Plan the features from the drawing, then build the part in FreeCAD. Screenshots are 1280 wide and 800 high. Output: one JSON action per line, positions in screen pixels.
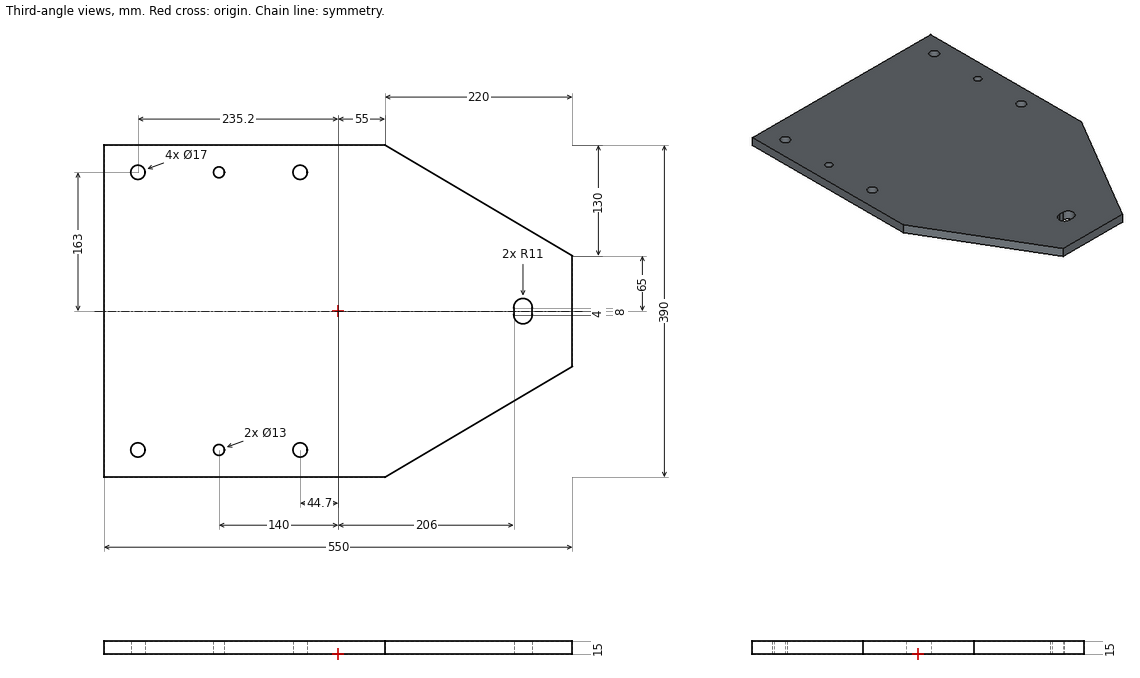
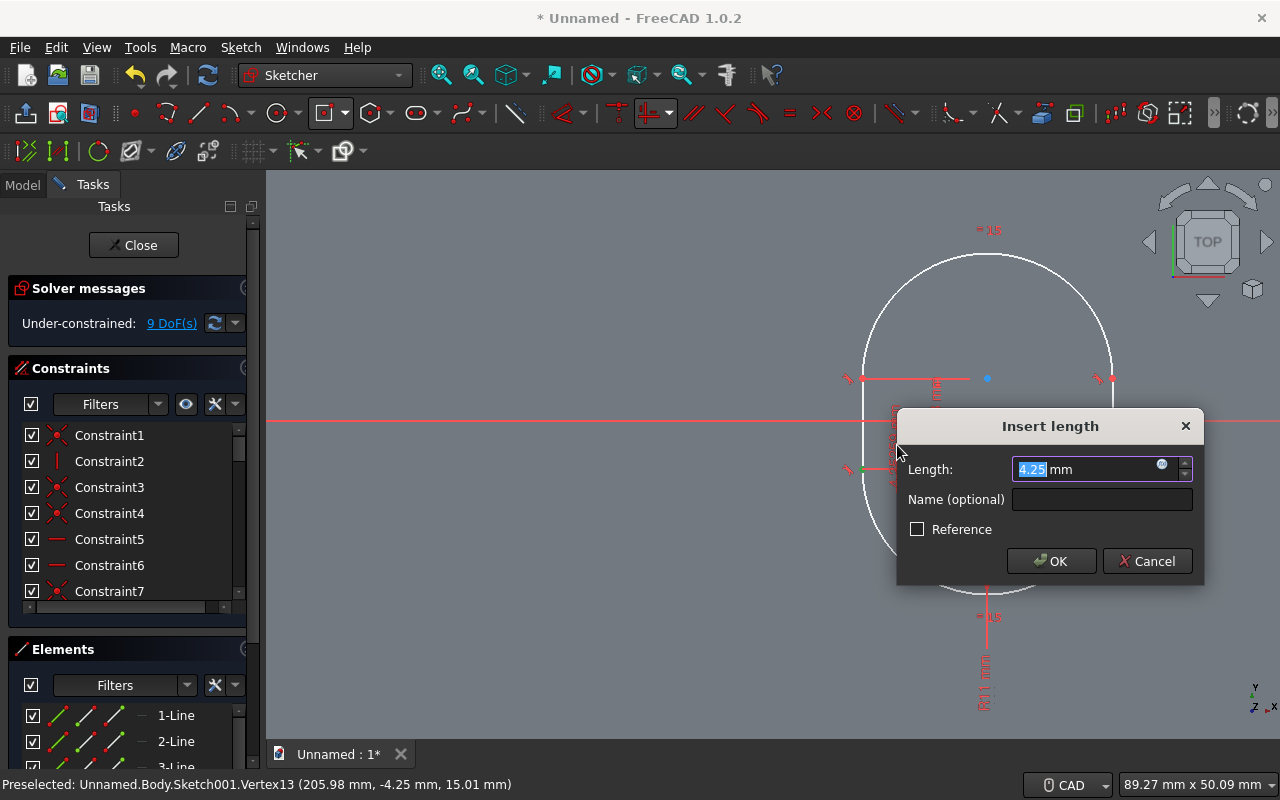
{"action": "type", "text": "4"}
{"action": "key", "text": "Return"}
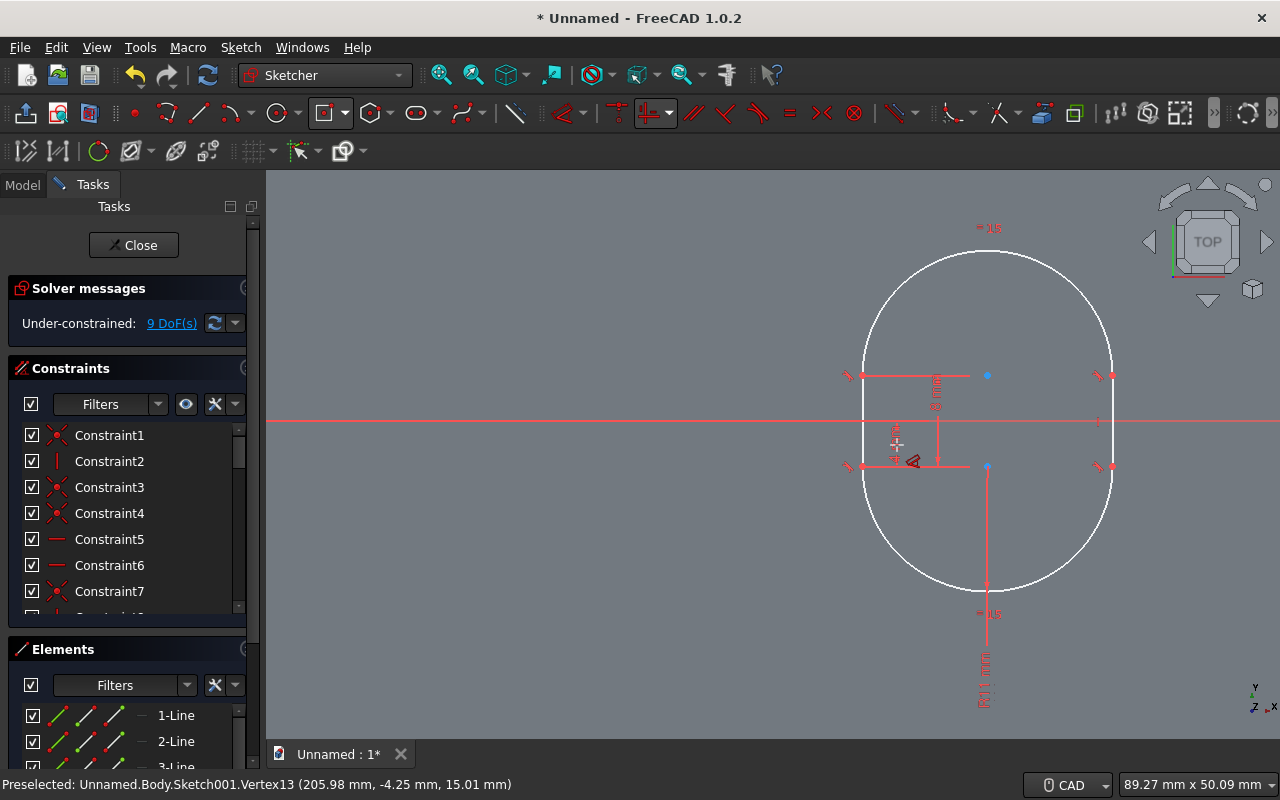
{"action": "scroll", "coordinate": [865, 457], "scroll_direction": "down", "scroll_amount": 13}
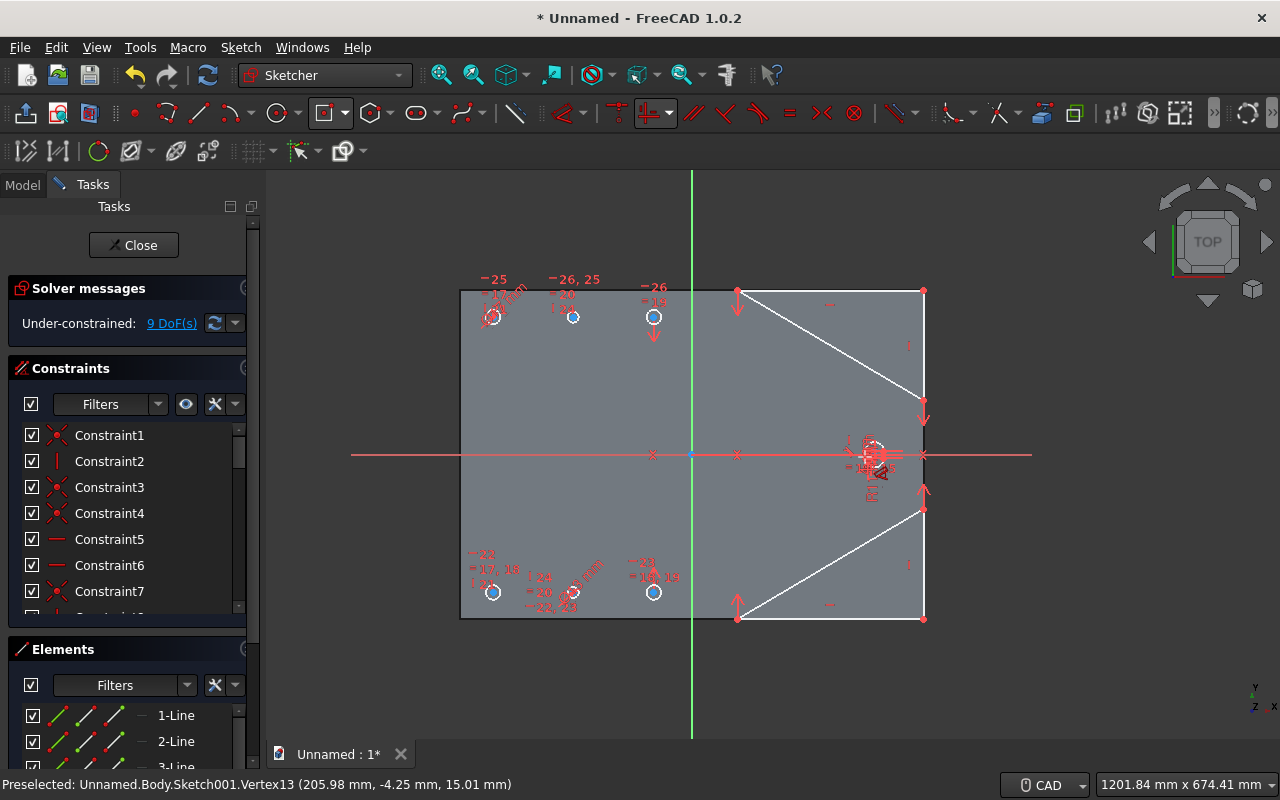
{"action": "left_click", "coordinate": [924, 368]}
{"action": "left_click", "coordinate": [958, 346]}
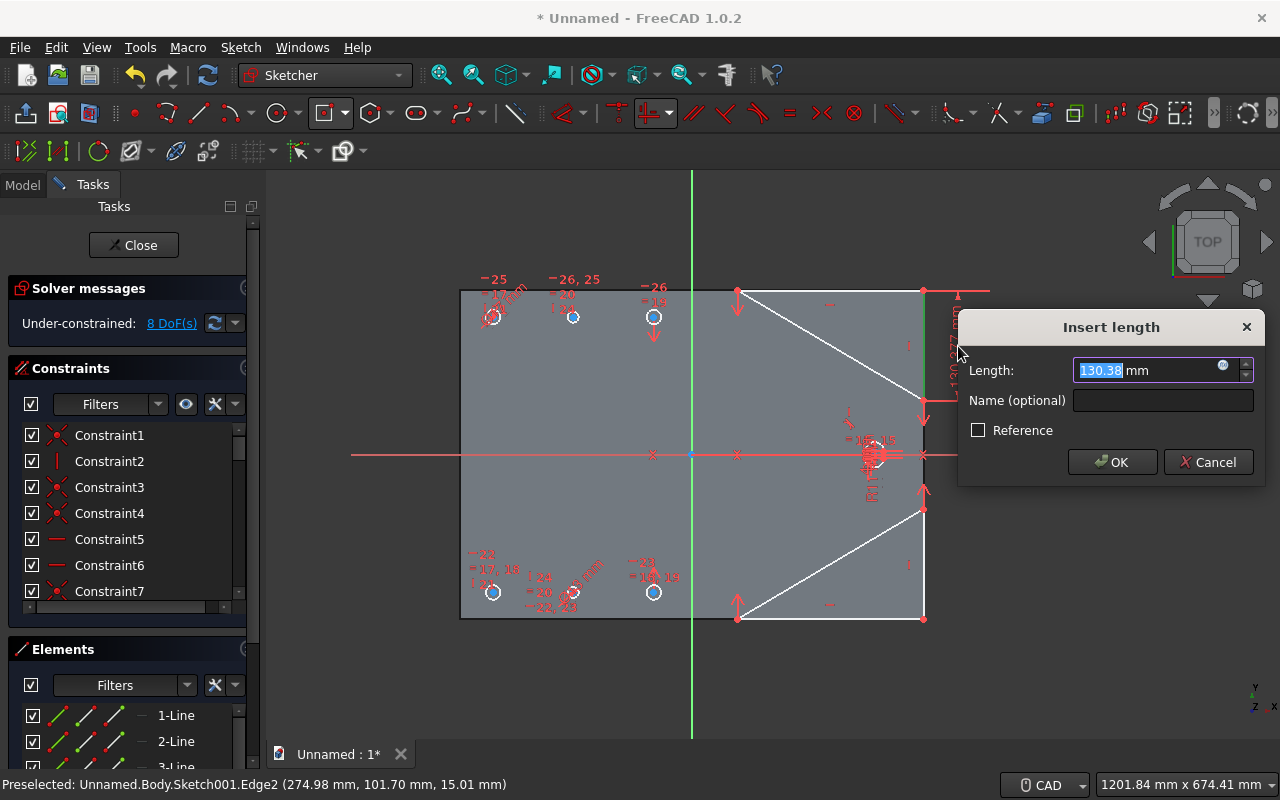
{"action": "type", "text": "130"}
{"action": "key", "text": "Return"}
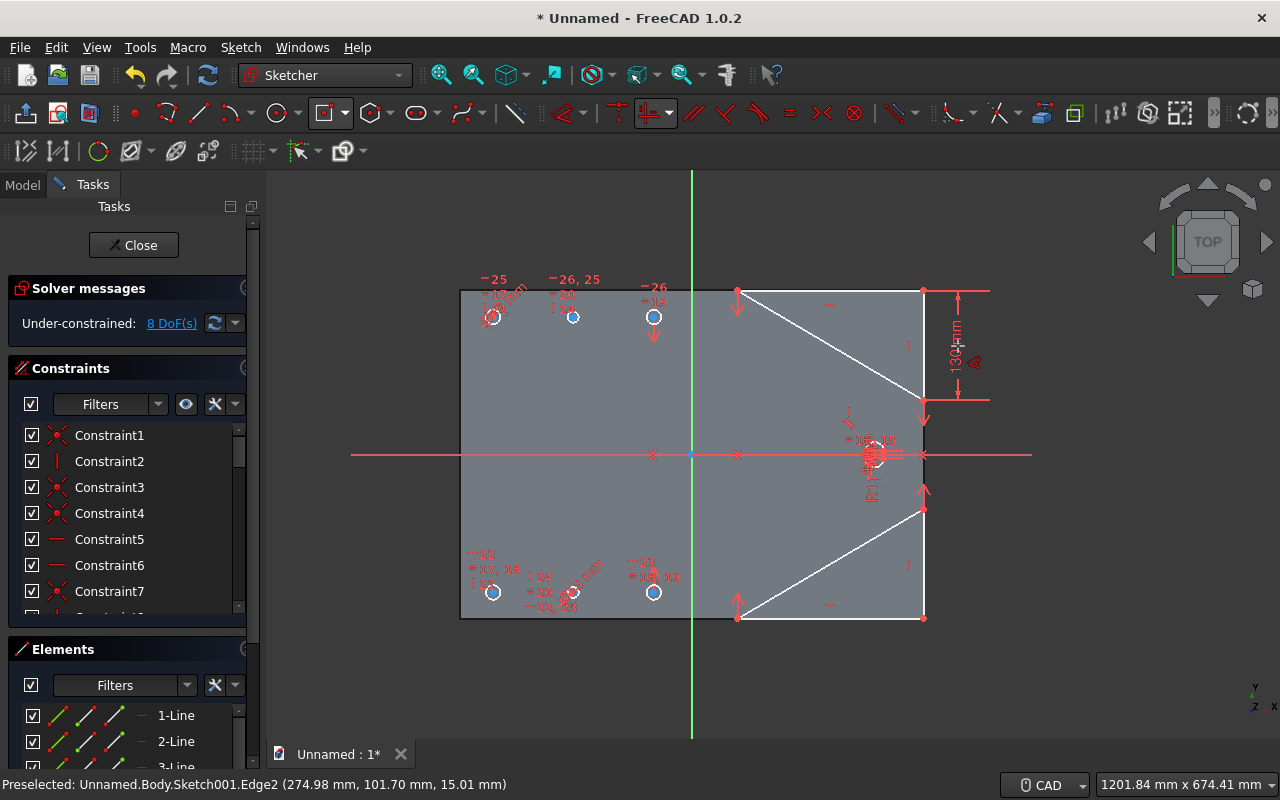
{"action": "left_click", "coordinate": [868, 291]}
{"action": "left_click", "coordinate": [831, 257]}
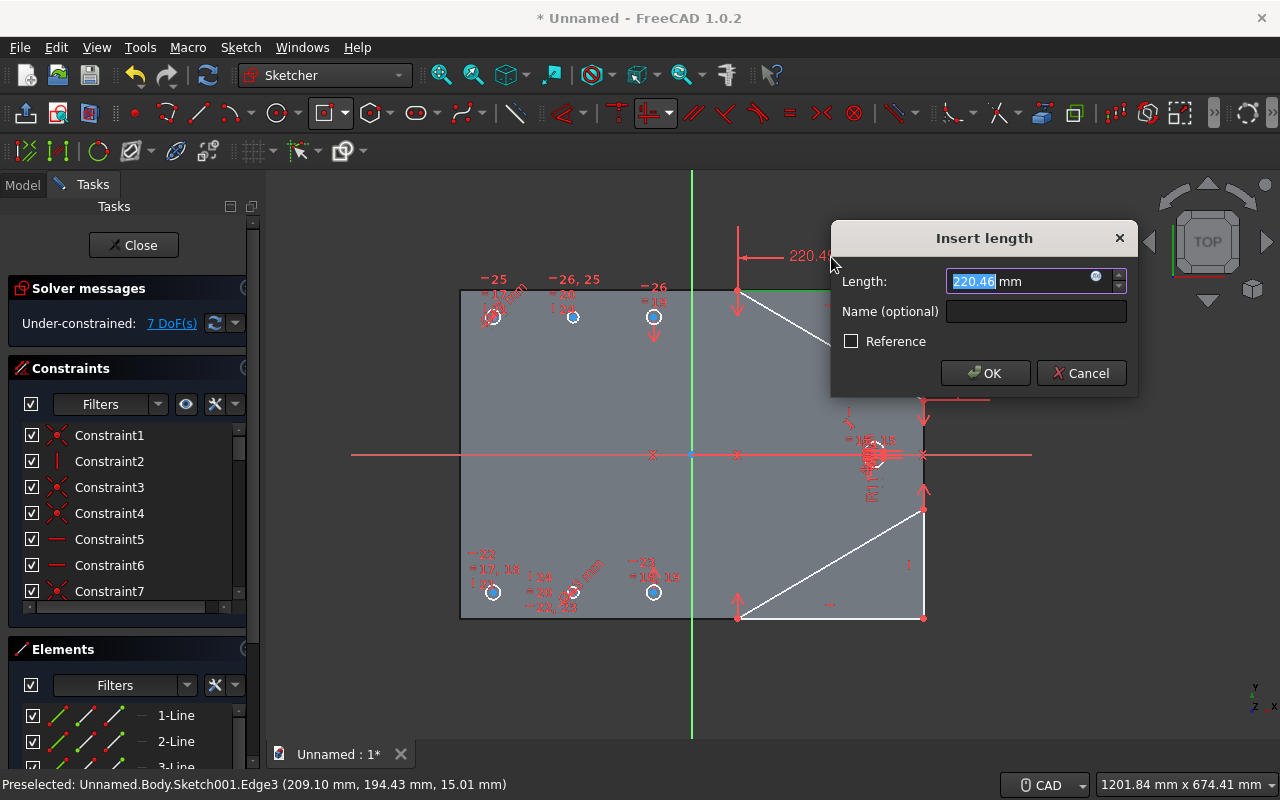
{"action": "type", "text": "220"}
{"action": "key", "text": "Return"}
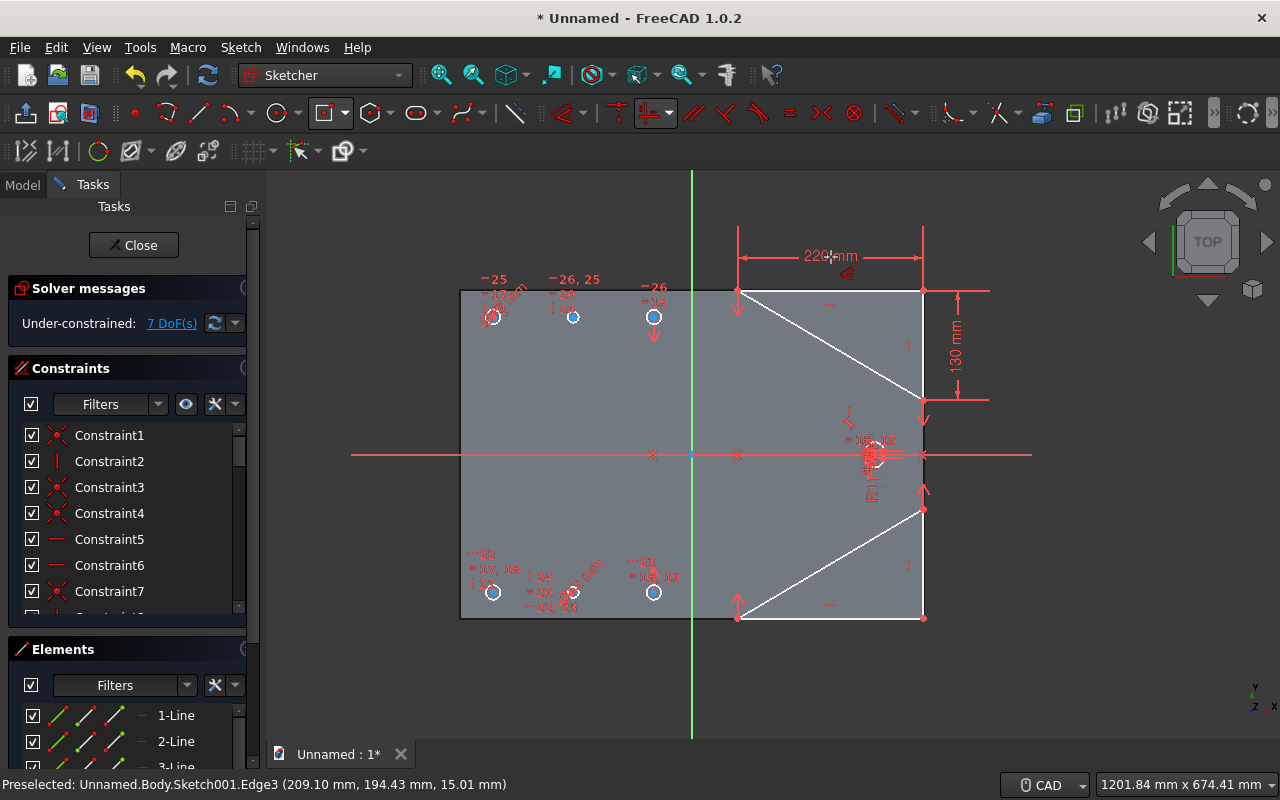
{"action": "left_click", "coordinate": [738, 291]}
{"action": "left_click", "coordinate": [715, 257]}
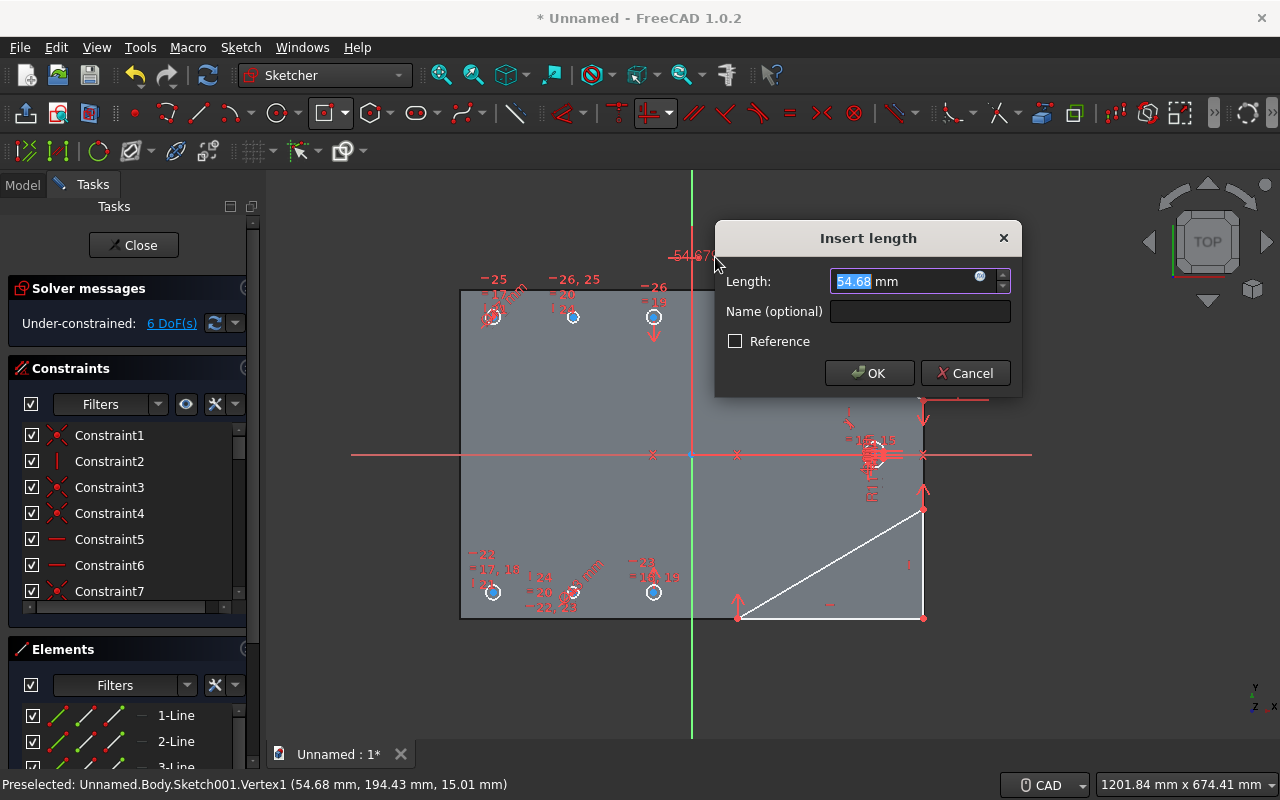
{"action": "type", "text": "55"}
{"action": "key", "text": "Return"}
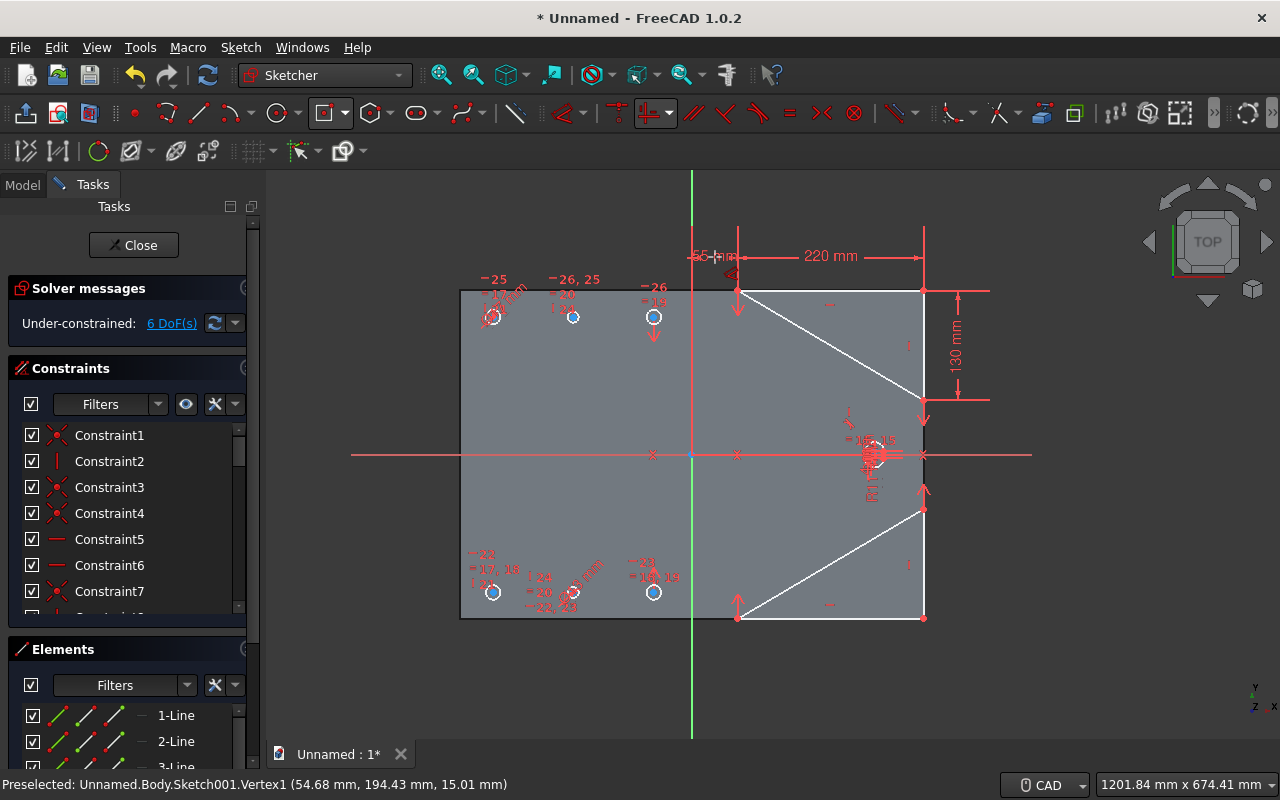
{"action": "left_click", "coordinate": [924, 400]}
{"action": "left_click", "coordinate": [958, 428]}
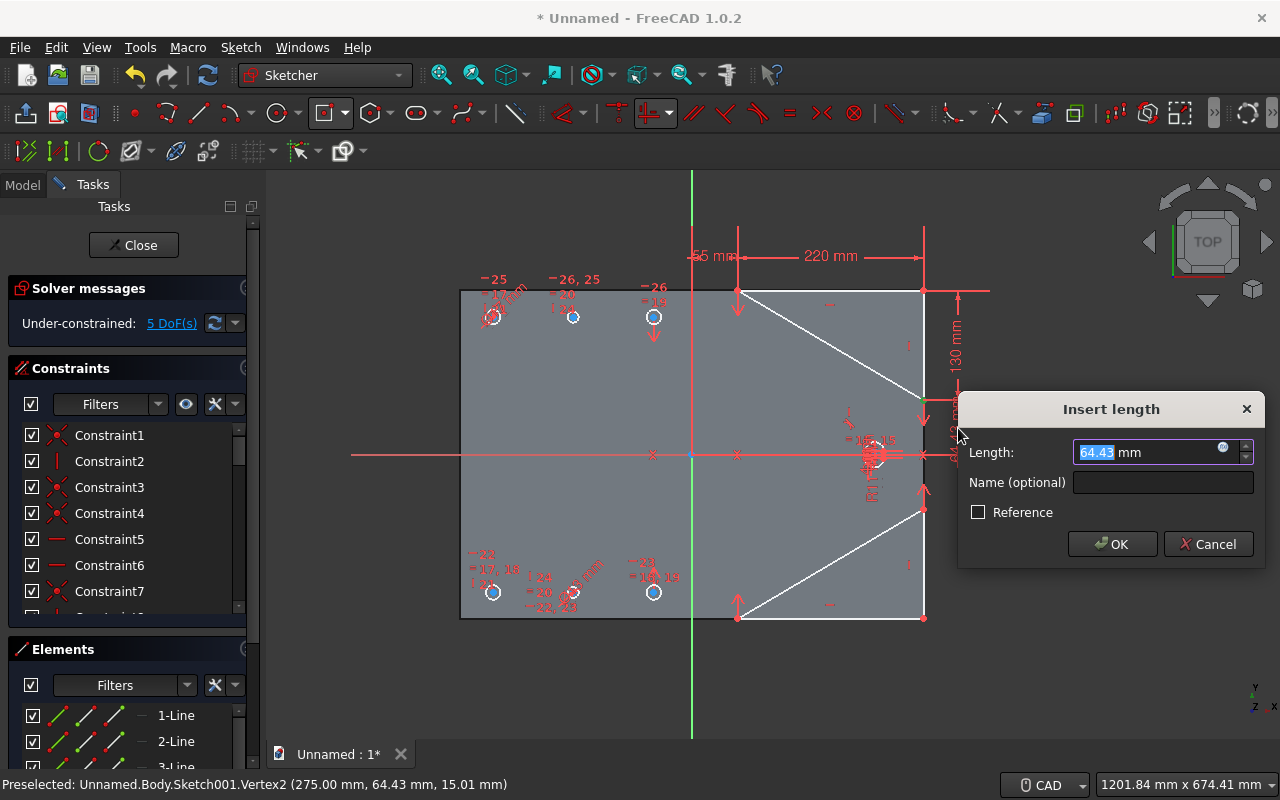
{"action": "type", "text": "65"}
{"action": "key", "text": "Return"}